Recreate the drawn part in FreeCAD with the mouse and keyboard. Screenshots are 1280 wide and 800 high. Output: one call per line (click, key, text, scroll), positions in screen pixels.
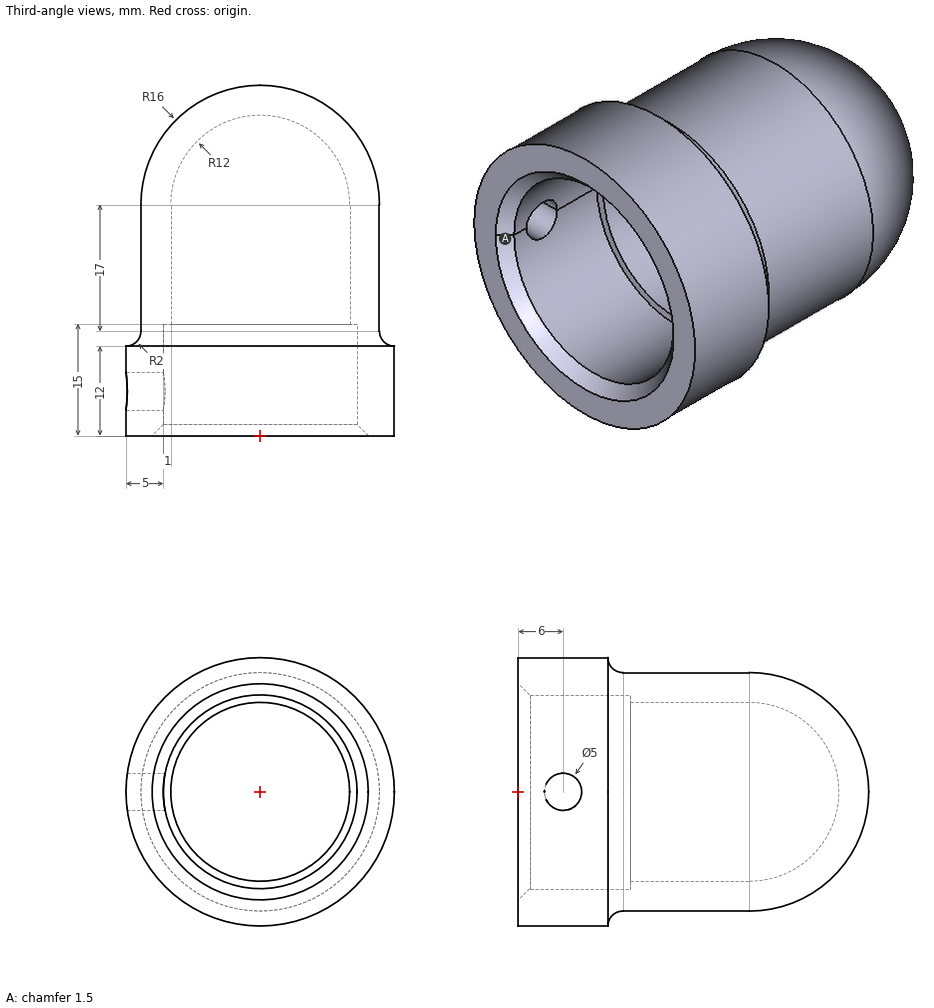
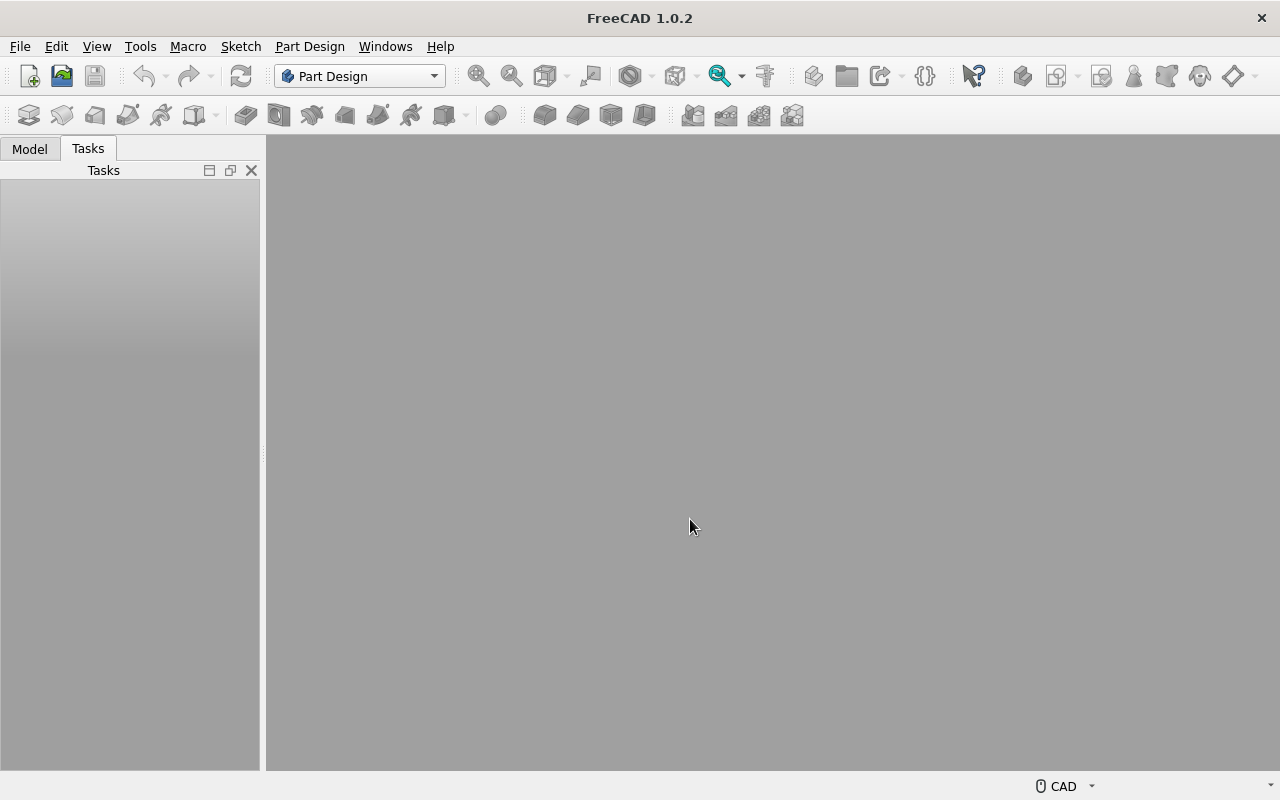
click(29, 76)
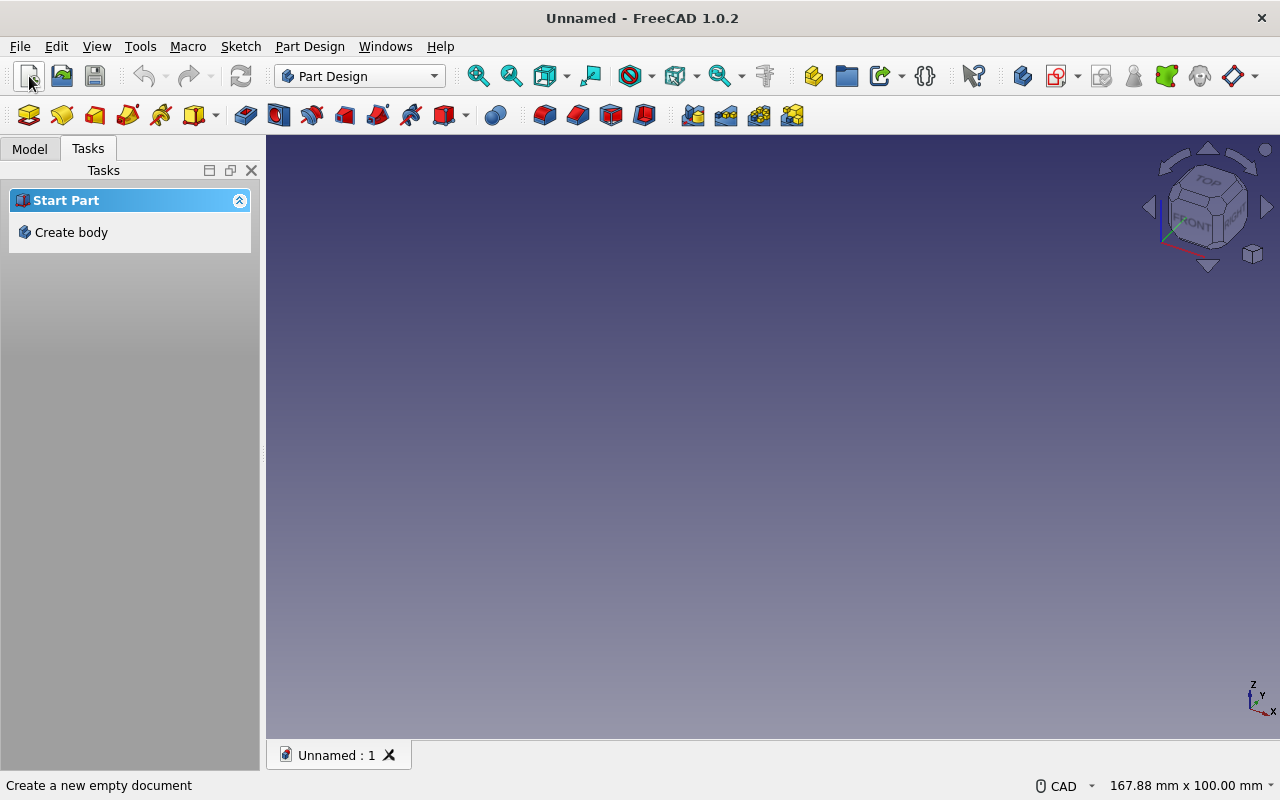
click(1056, 76)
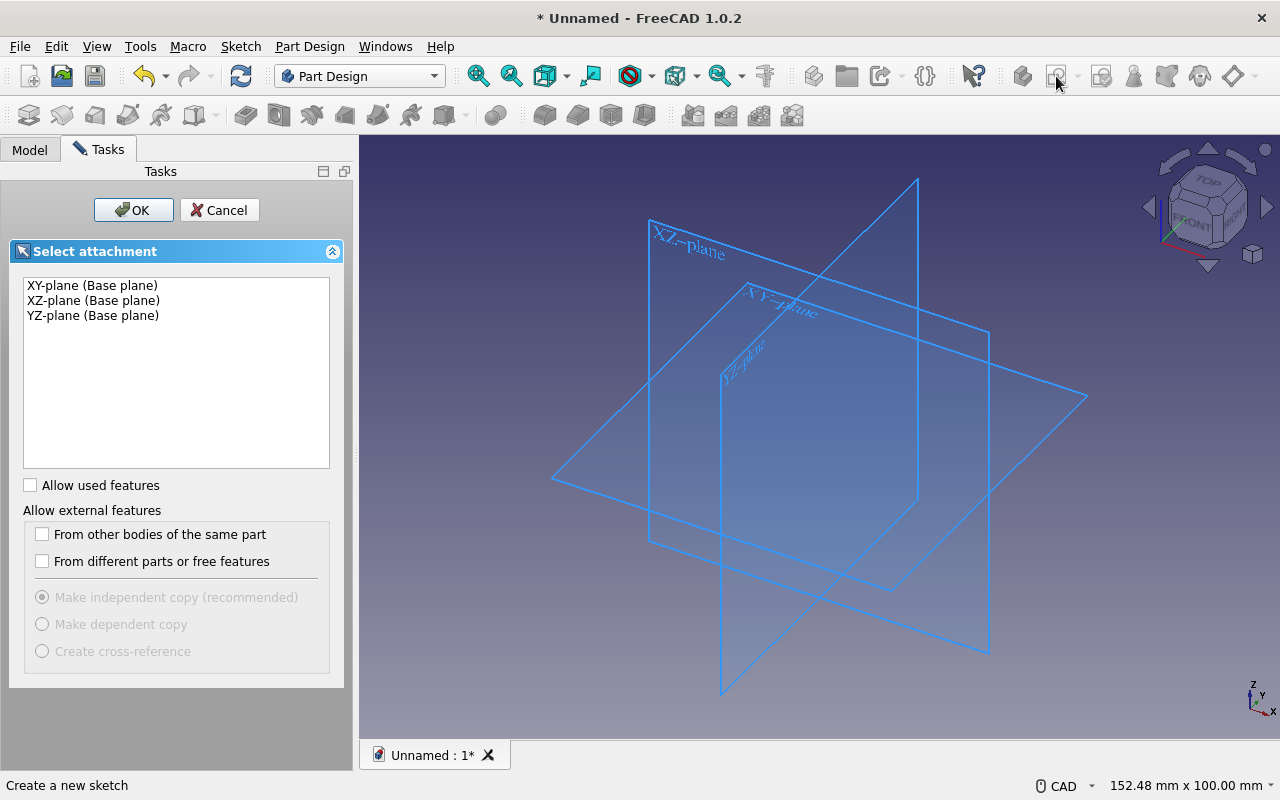
click(84, 286)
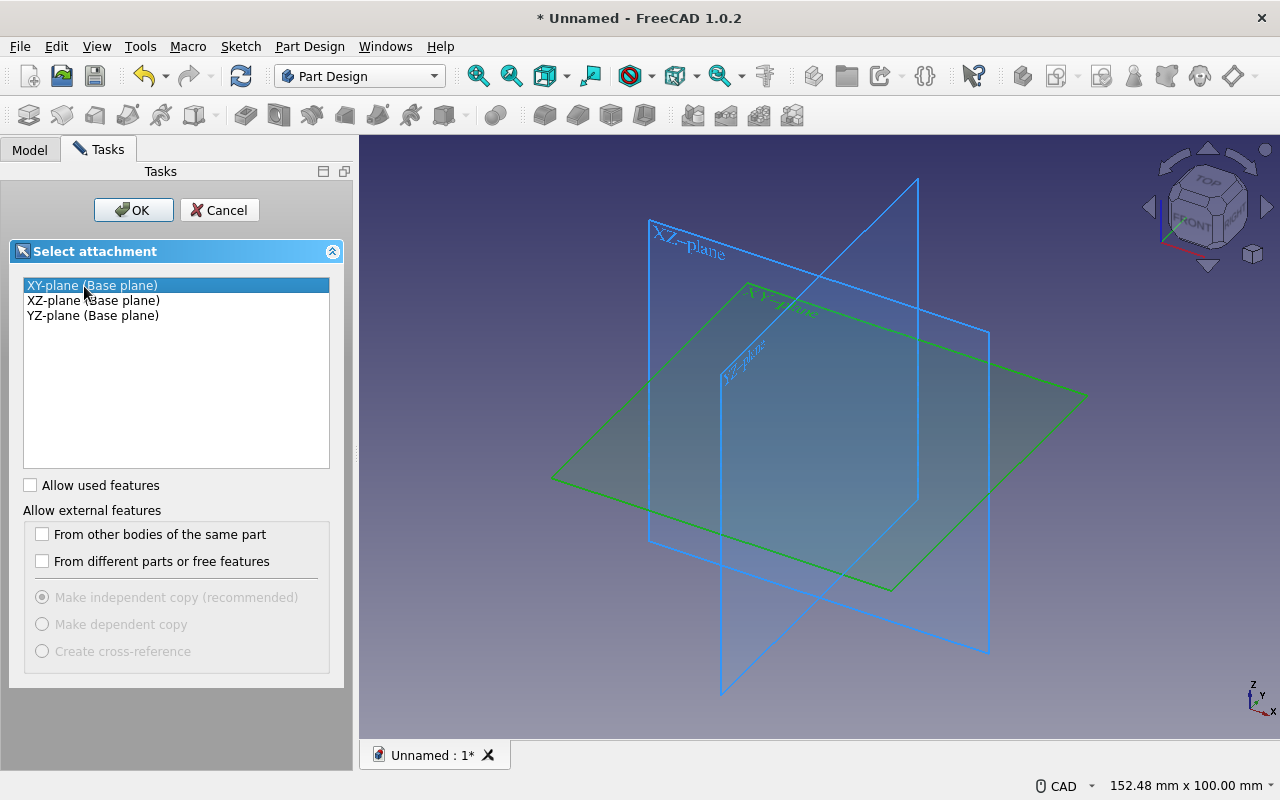
click(134, 210)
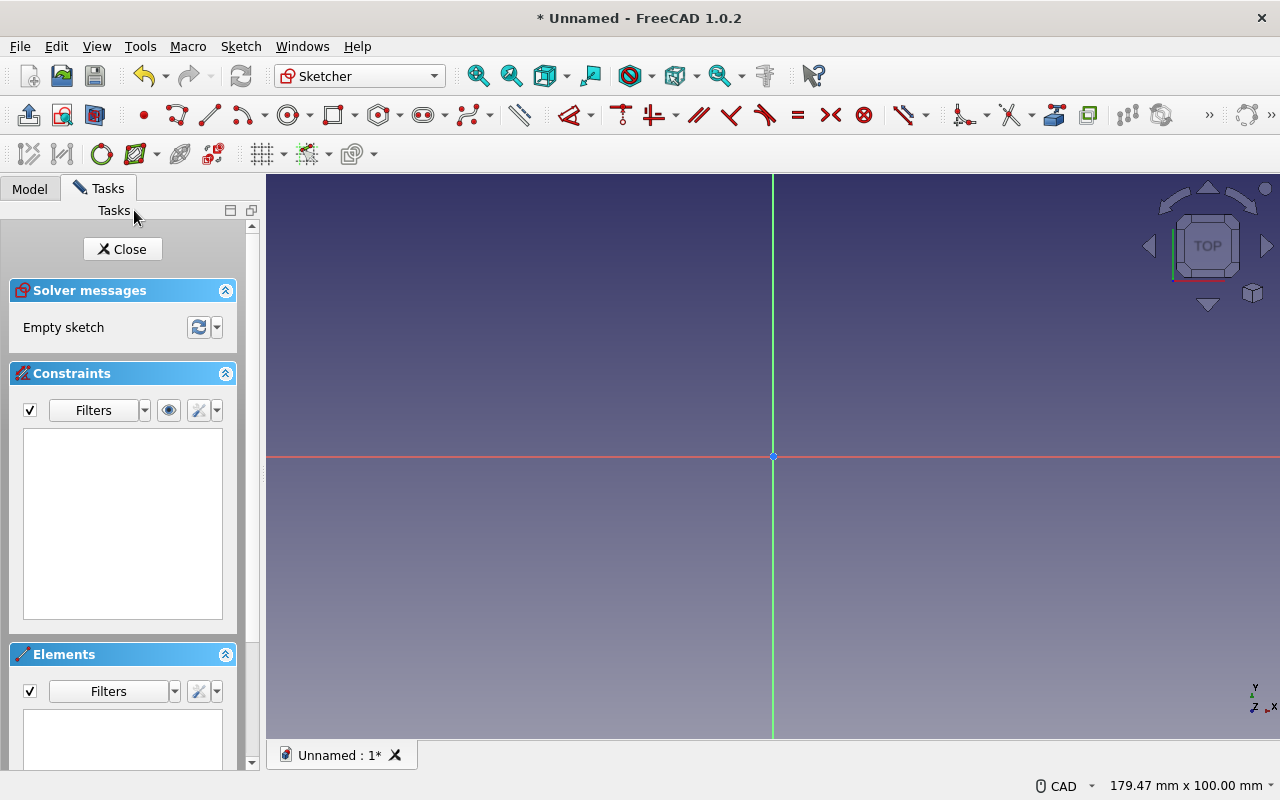
scroll(625, 711, down, 1)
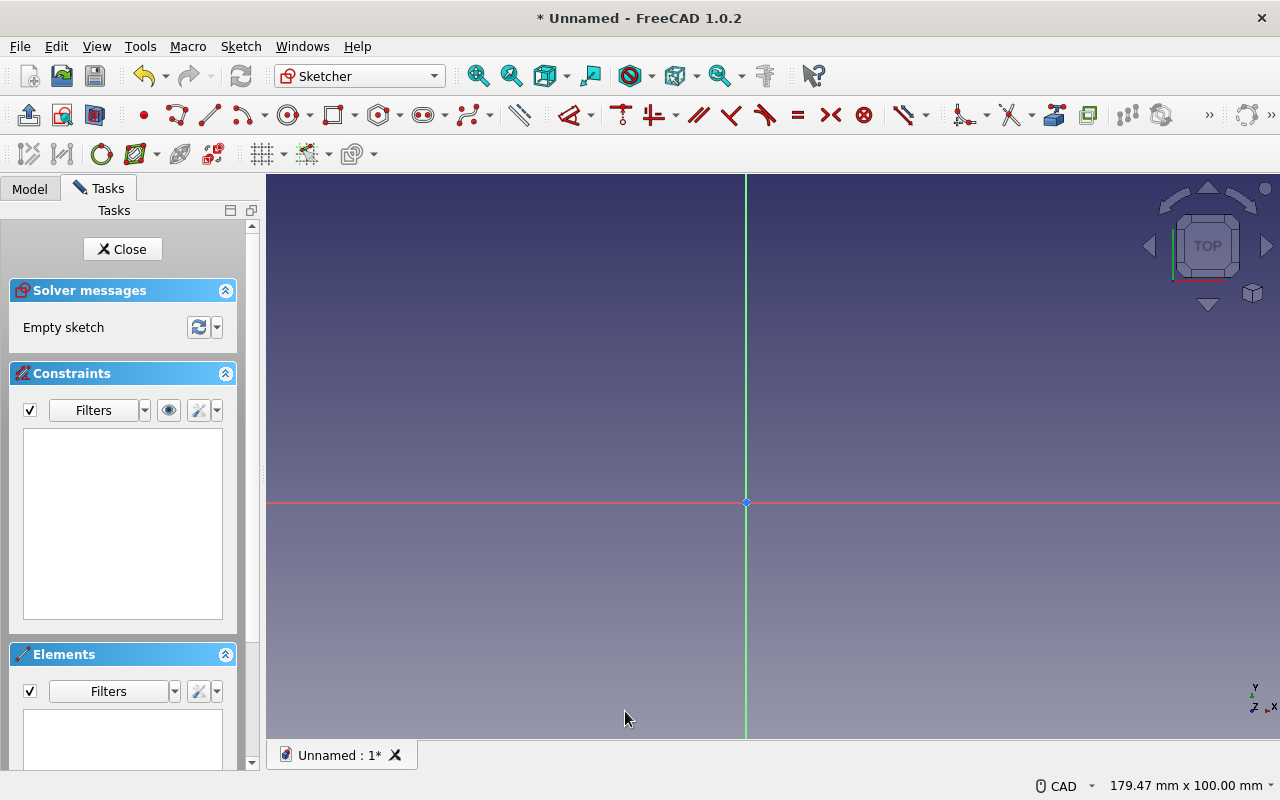
scroll(705, 318, up, 3)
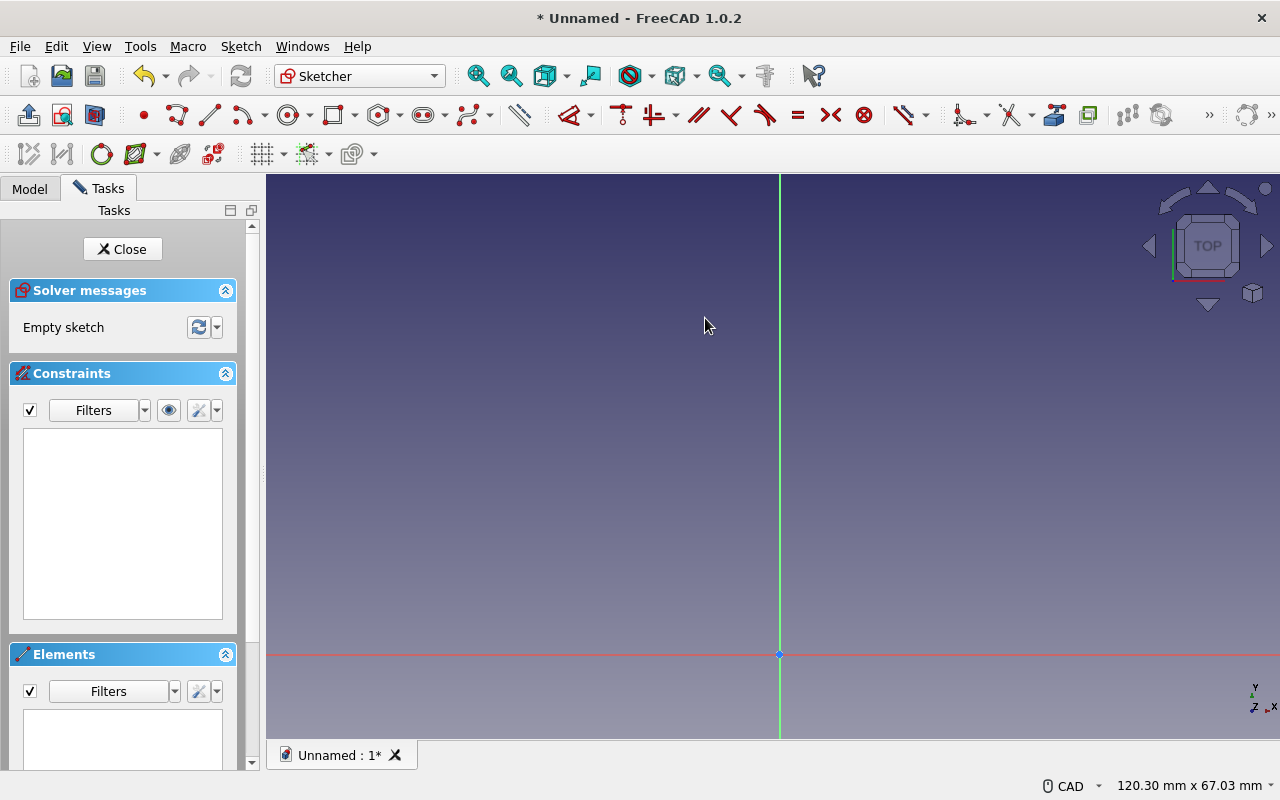
click(210, 116)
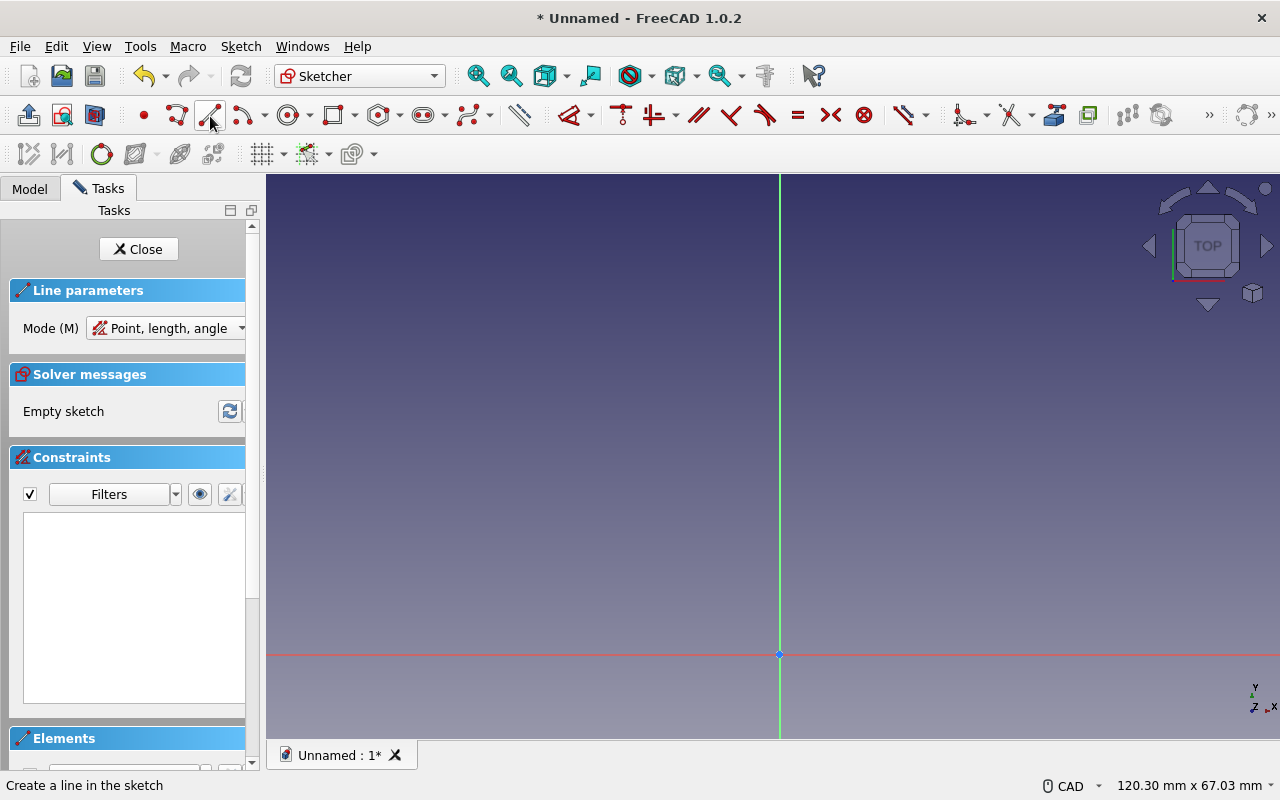
click(645, 393)
click(645, 537)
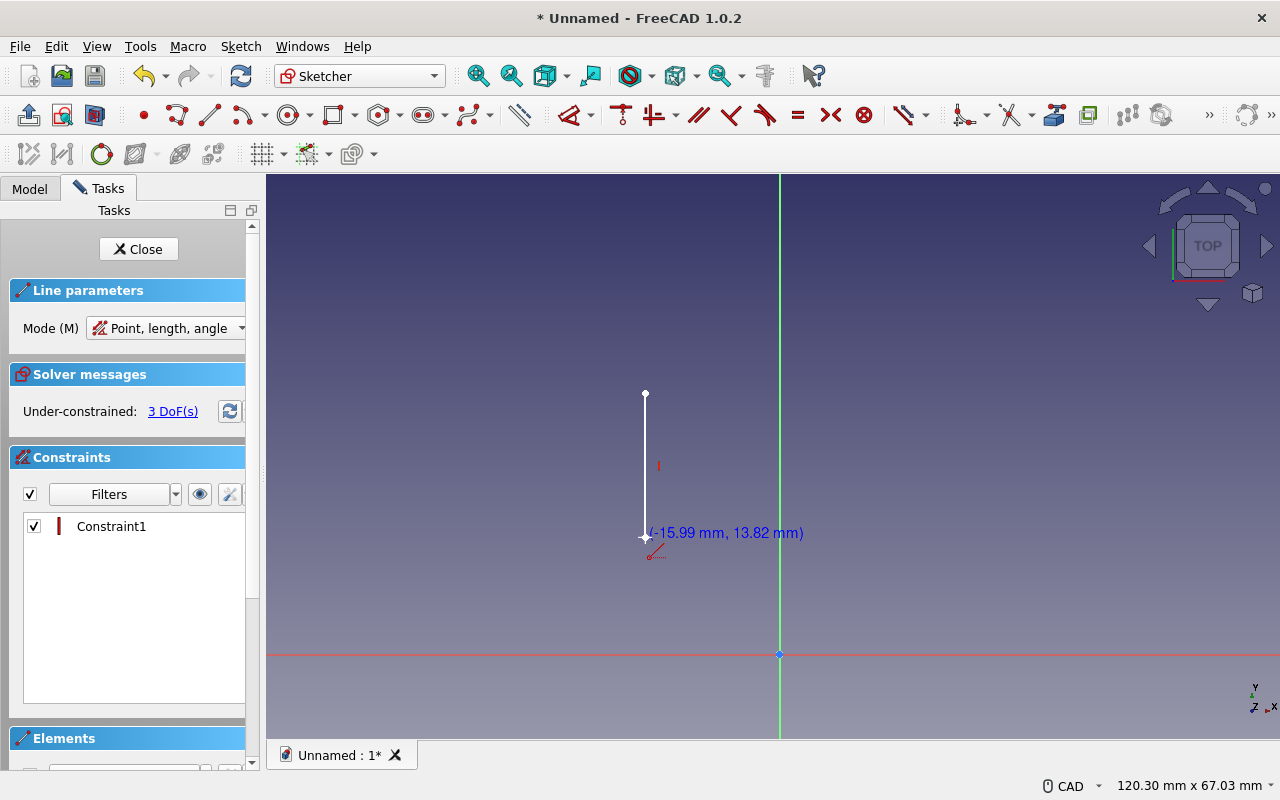
click(177, 116)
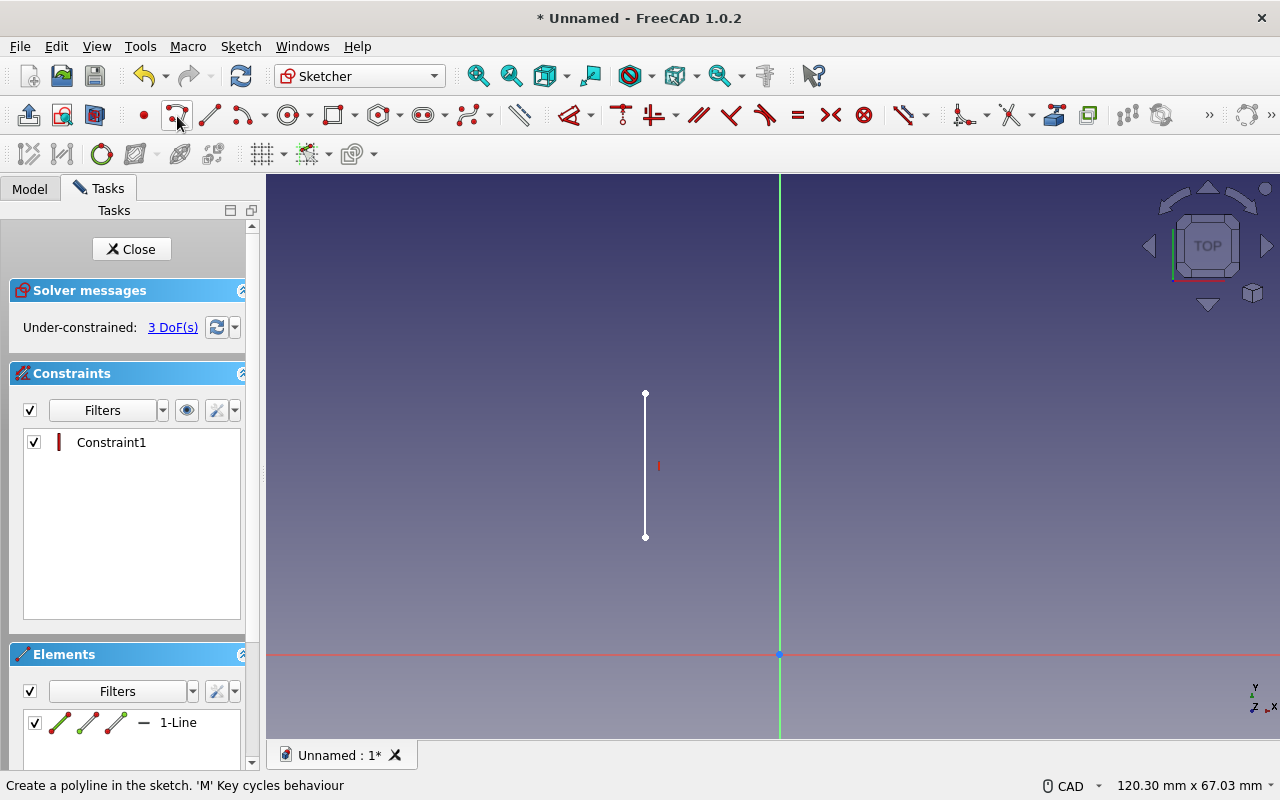
click(628, 553)
click(628, 655)
click(670, 646)
click(670, 528)